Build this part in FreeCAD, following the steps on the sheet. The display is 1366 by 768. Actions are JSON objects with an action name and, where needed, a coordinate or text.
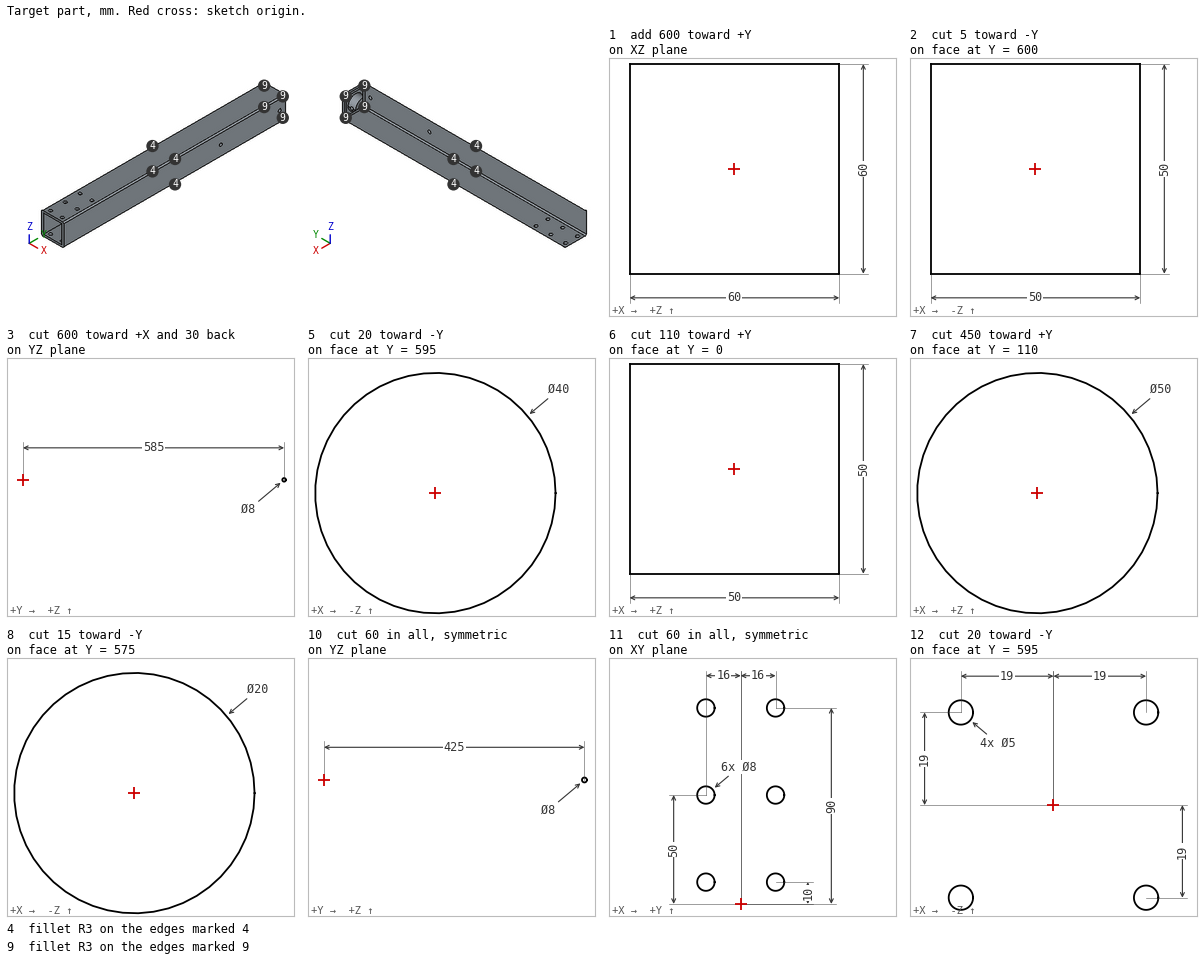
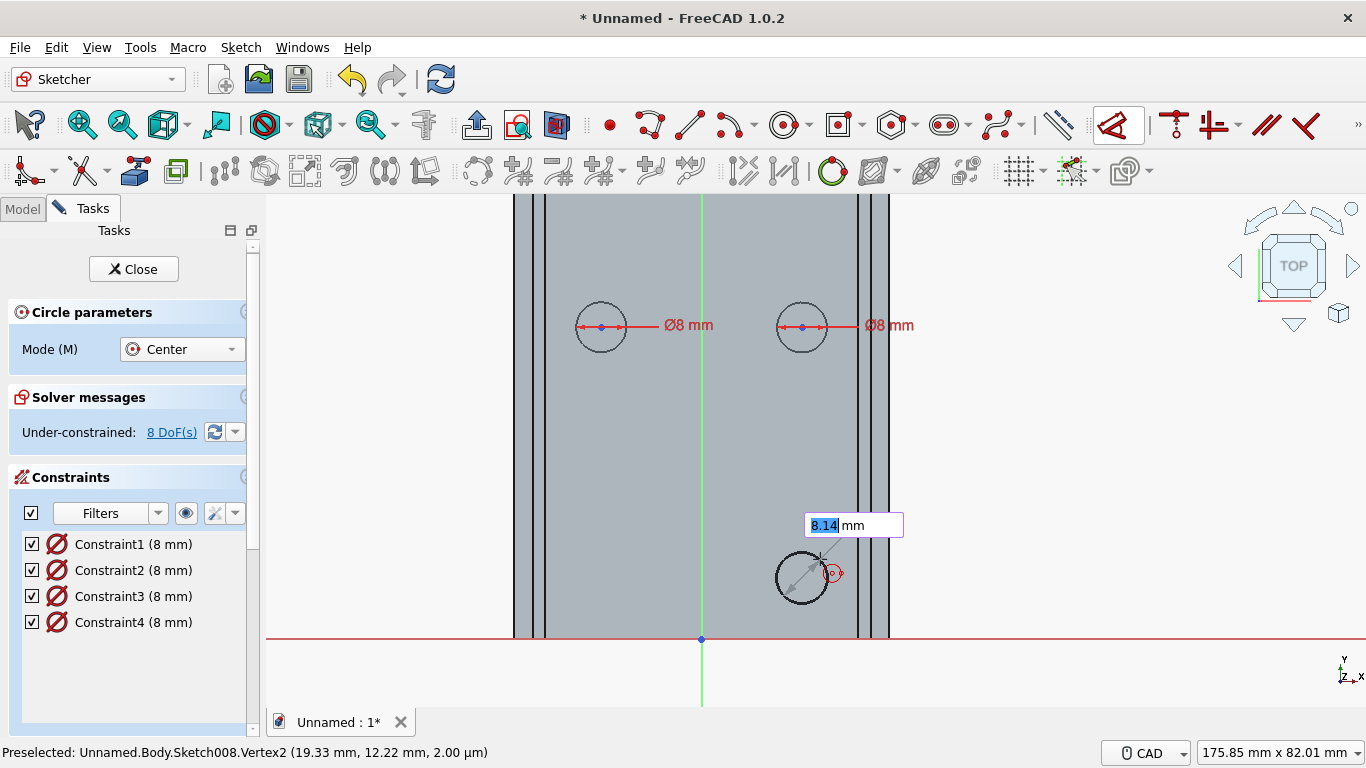
{"action": "type", "text": "8"}
{"action": "key", "text": "Return"}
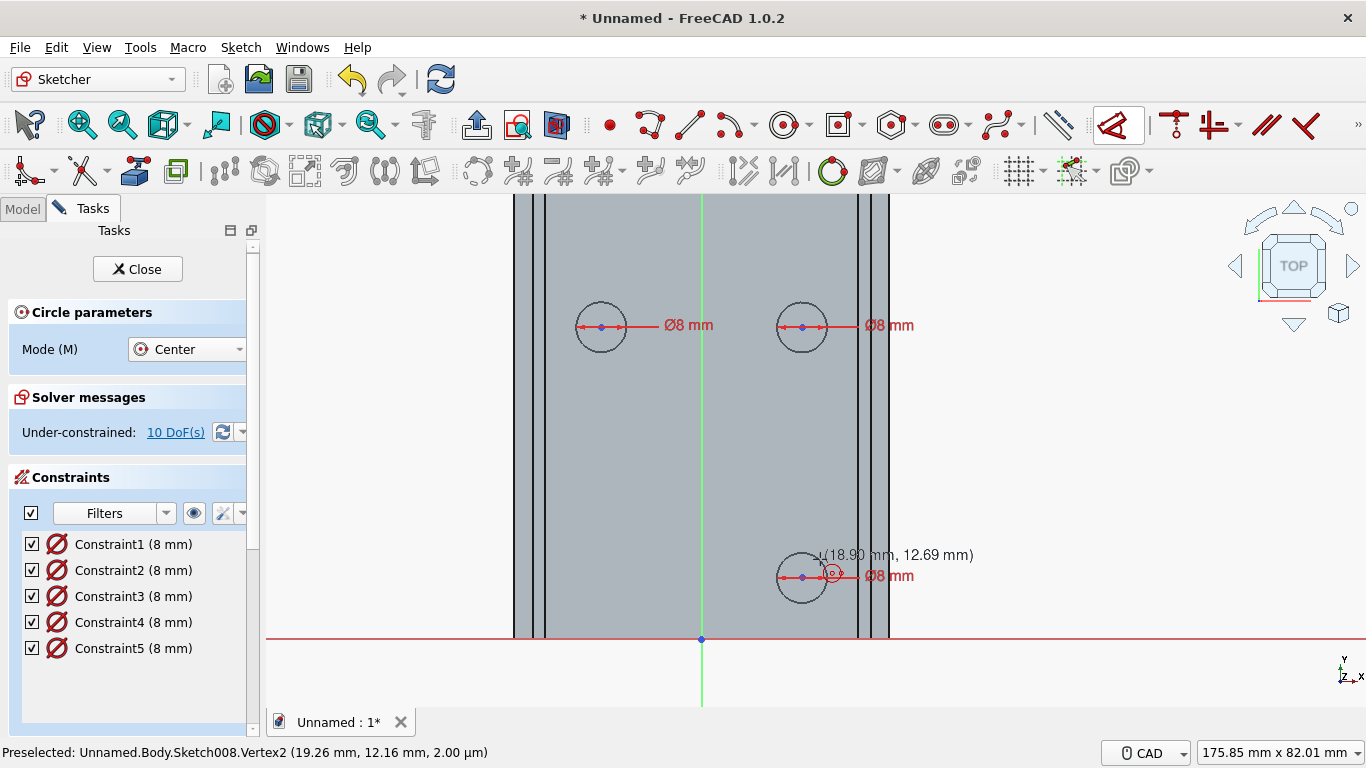
{"action": "left_click", "coordinate": [602, 577]}
{"action": "mouse_move", "coordinate": [619, 559]}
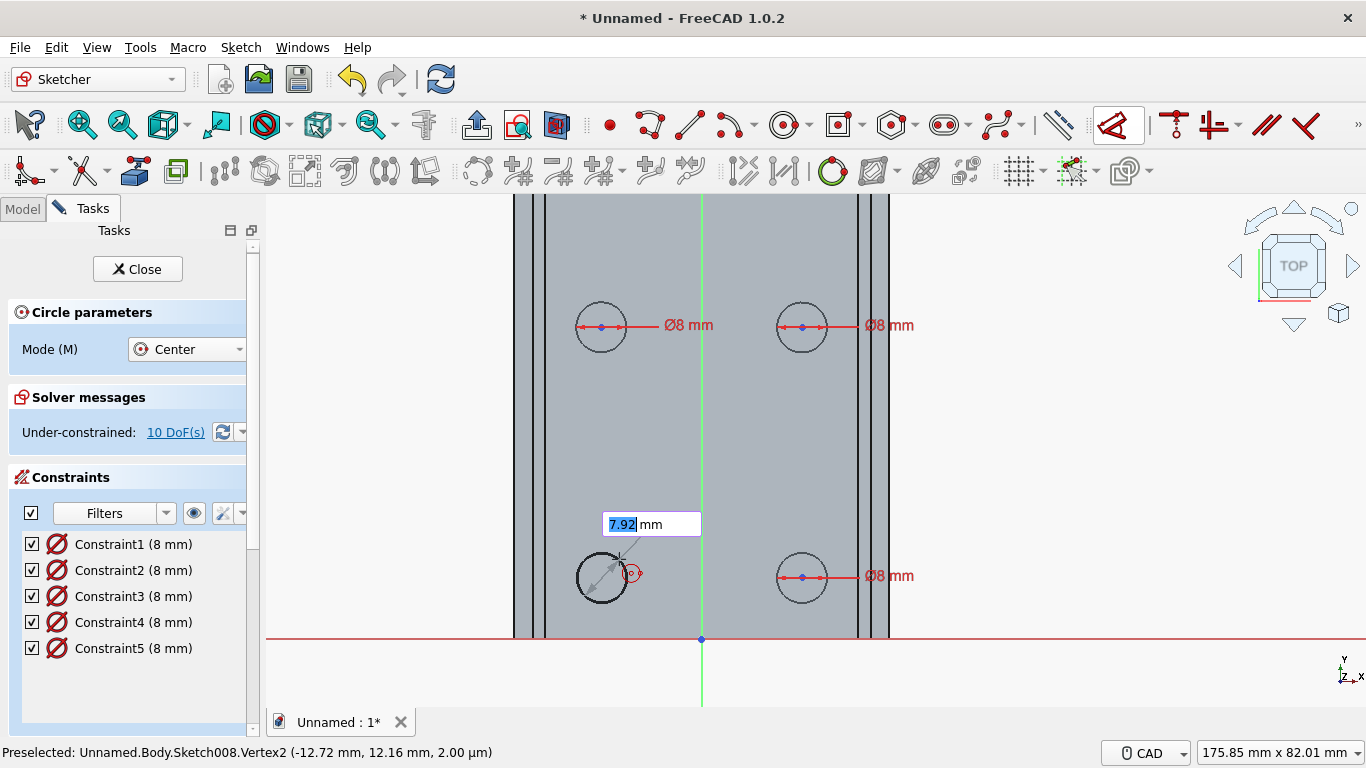
{"action": "type", "text": "8"}
{"action": "key", "text": "Return"}
{"action": "key", "text": "Escape"}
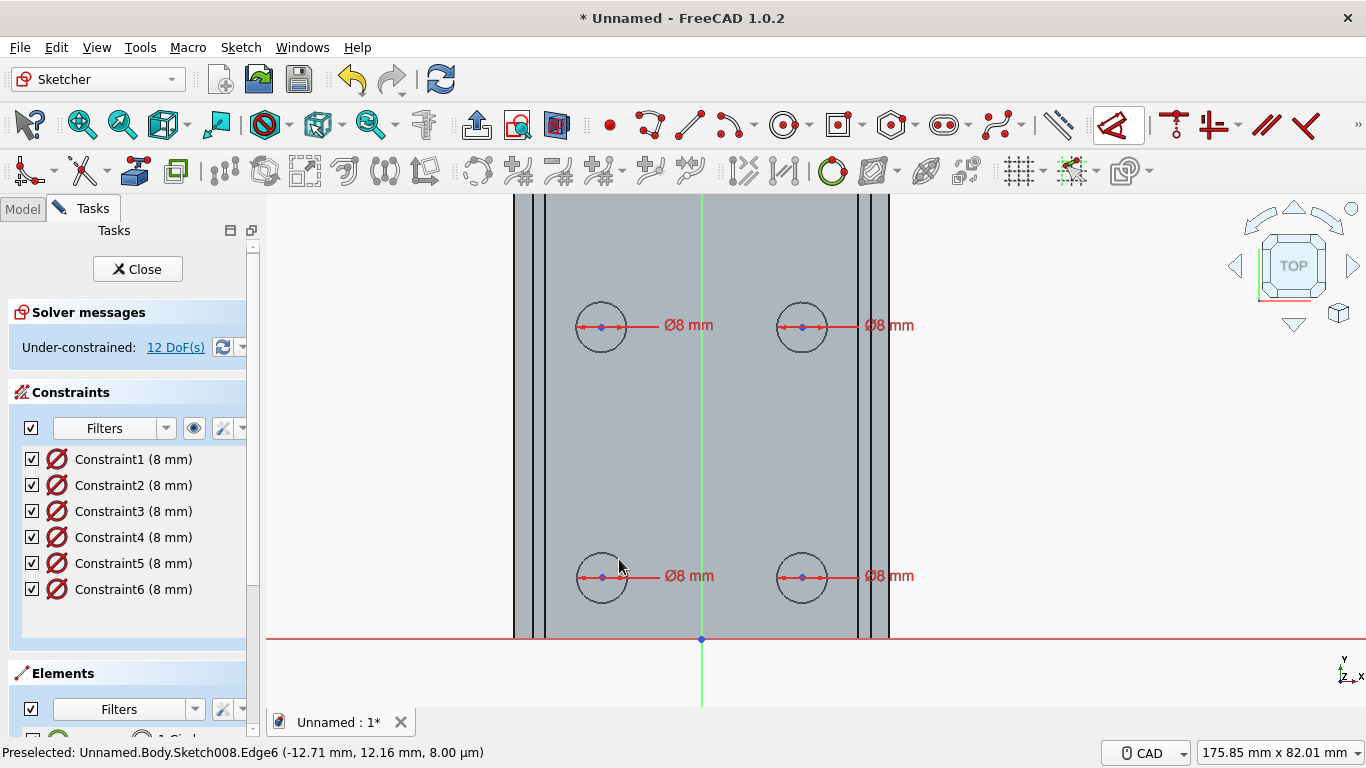
{"action": "scroll", "coordinate": [803, 578], "scroll_direction": "down", "scroll_amount": 3}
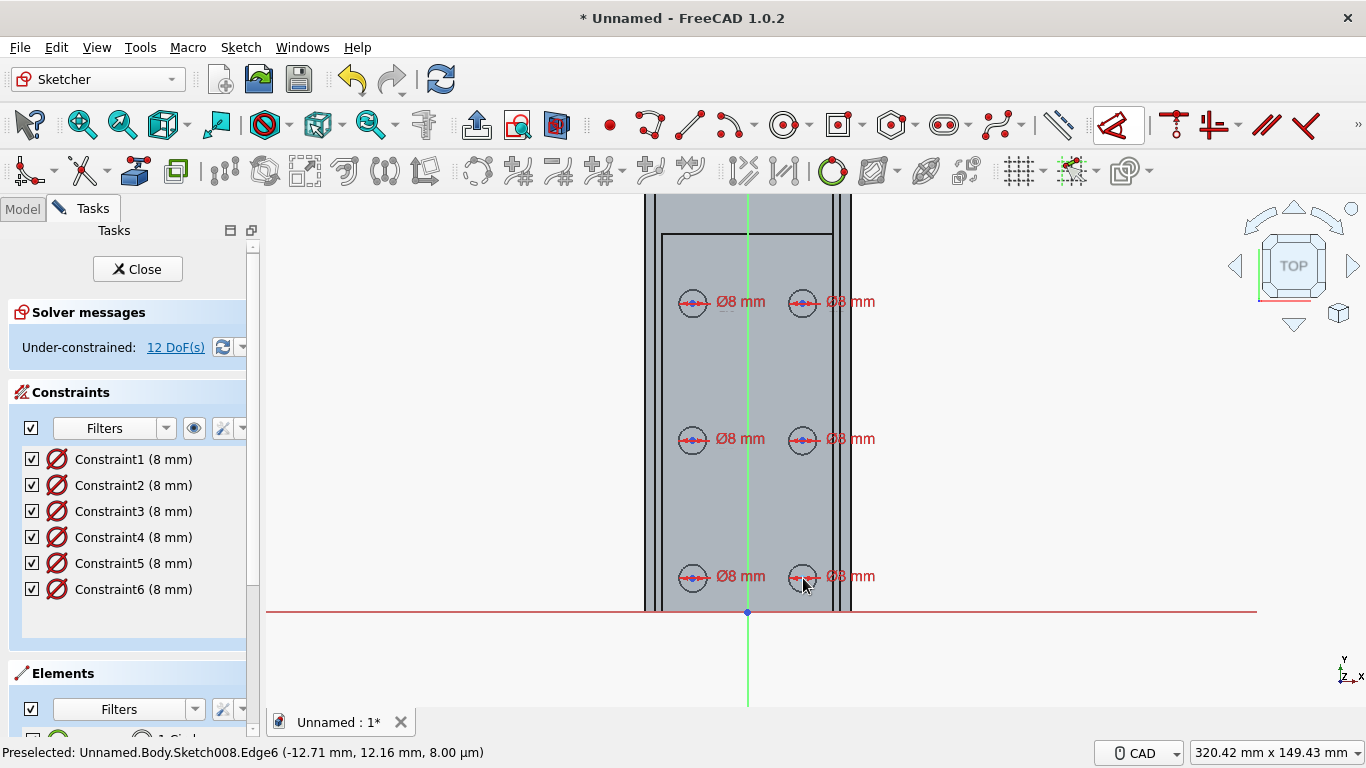
{"action": "left_click", "coordinate": [803, 304]}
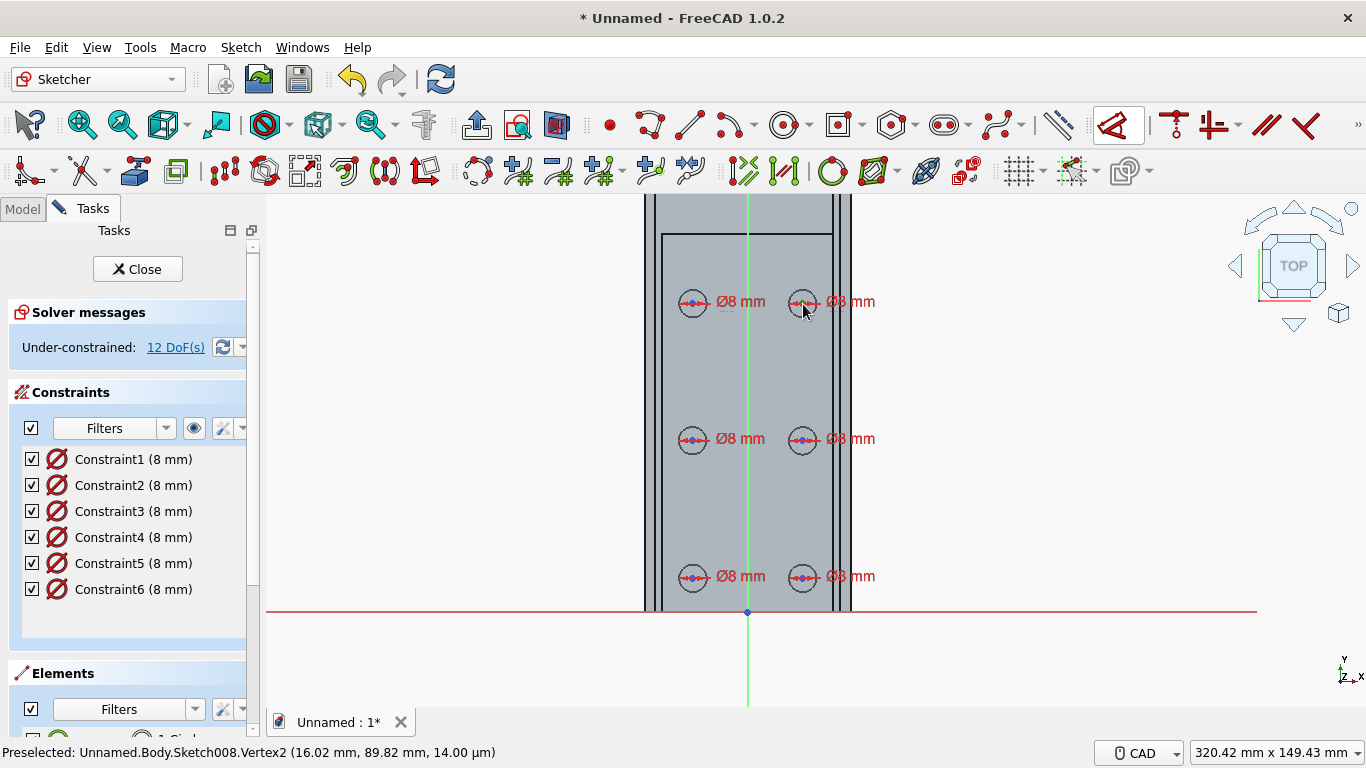
{"action": "left_click", "coordinate": [803, 441]}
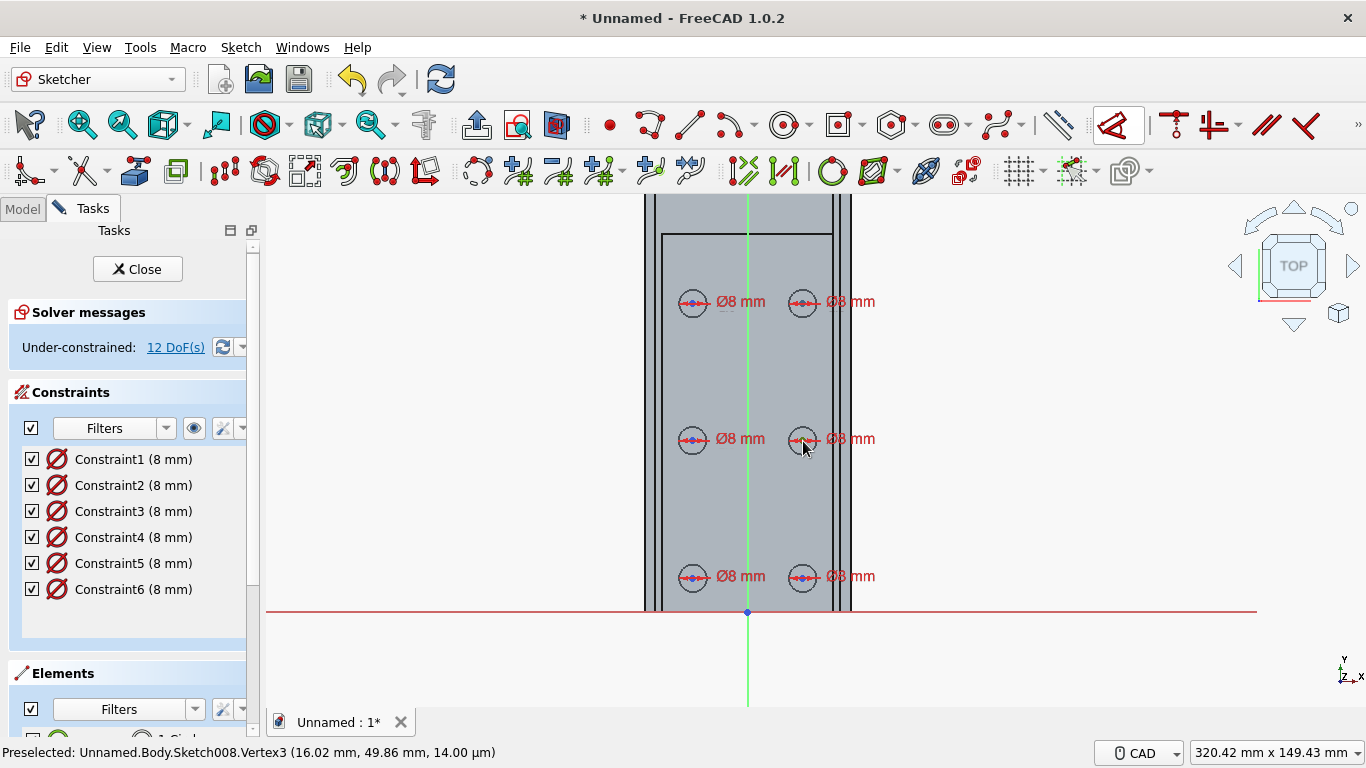
{"action": "key", "text": "v"}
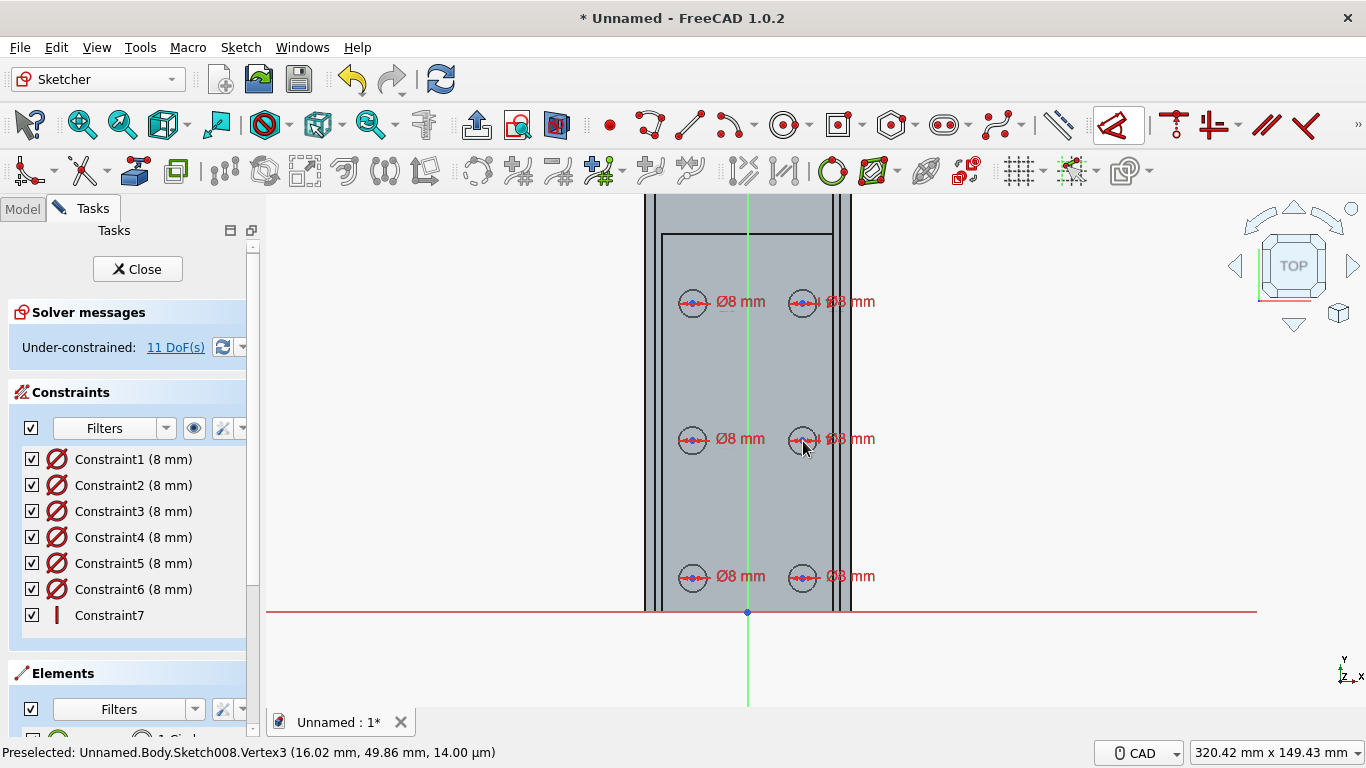
{"action": "left_click", "coordinate": [692, 441]}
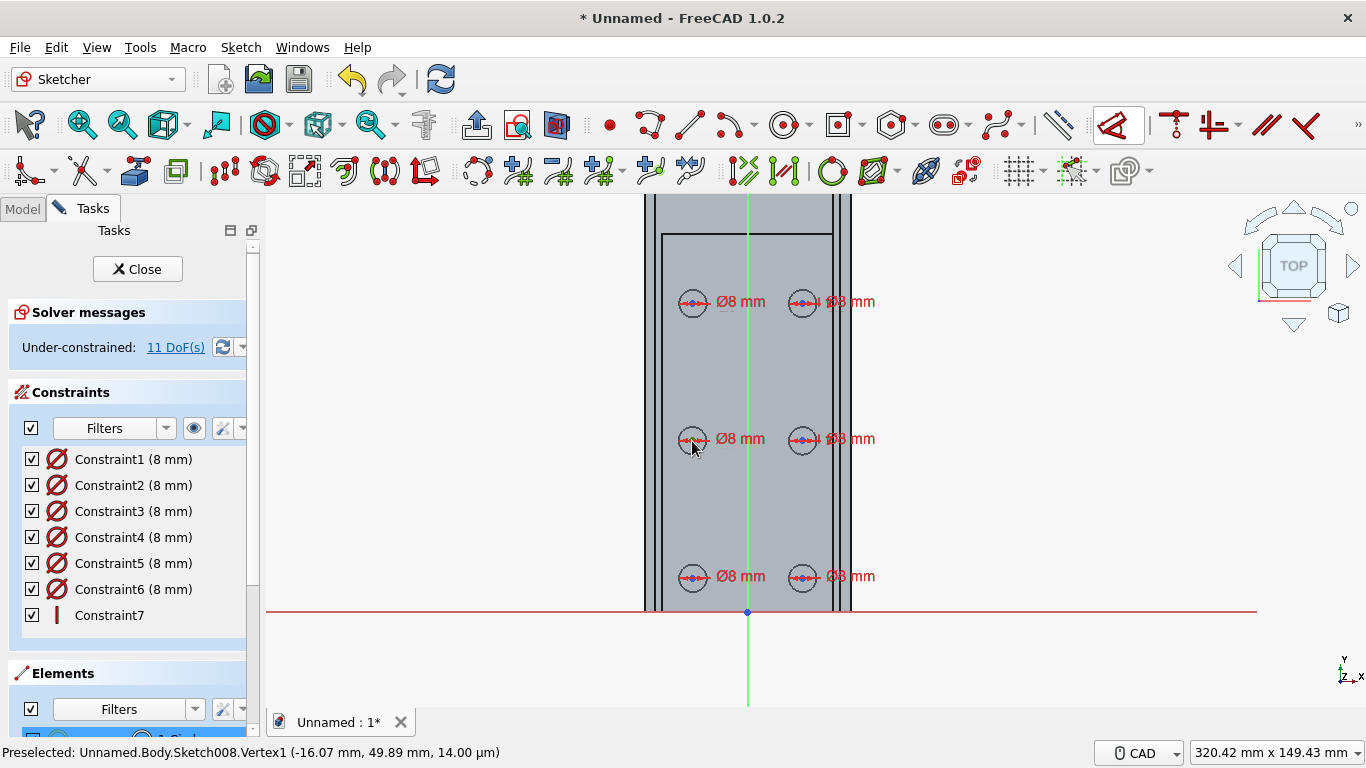
{"action": "left_click", "coordinate": [803, 441]}